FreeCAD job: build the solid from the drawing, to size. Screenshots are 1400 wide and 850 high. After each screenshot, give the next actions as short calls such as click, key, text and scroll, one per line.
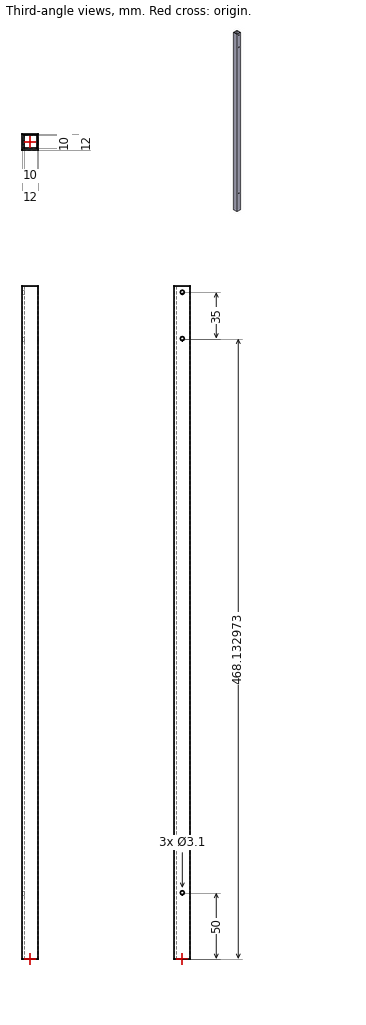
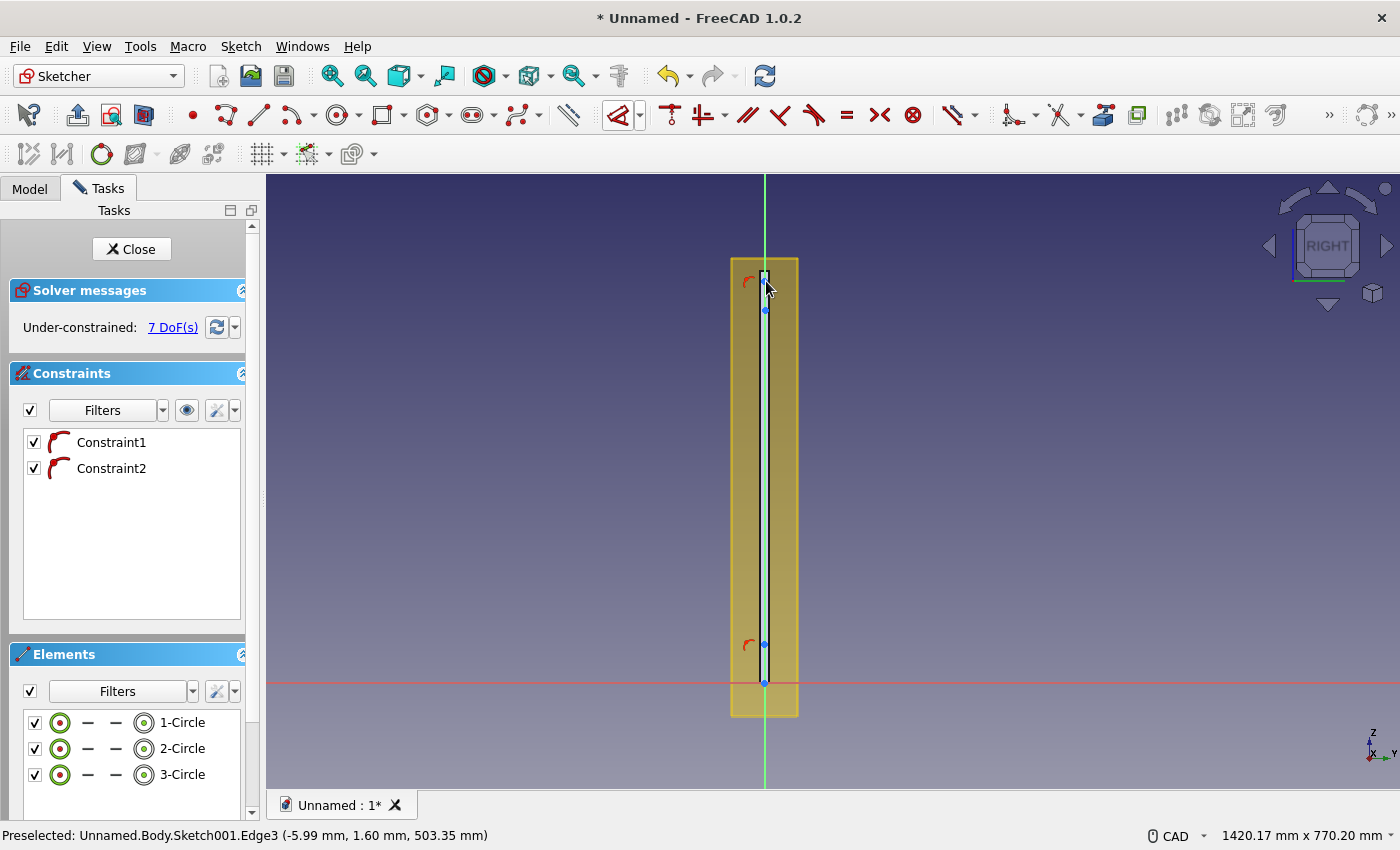
scroll(766, 643, up, 13)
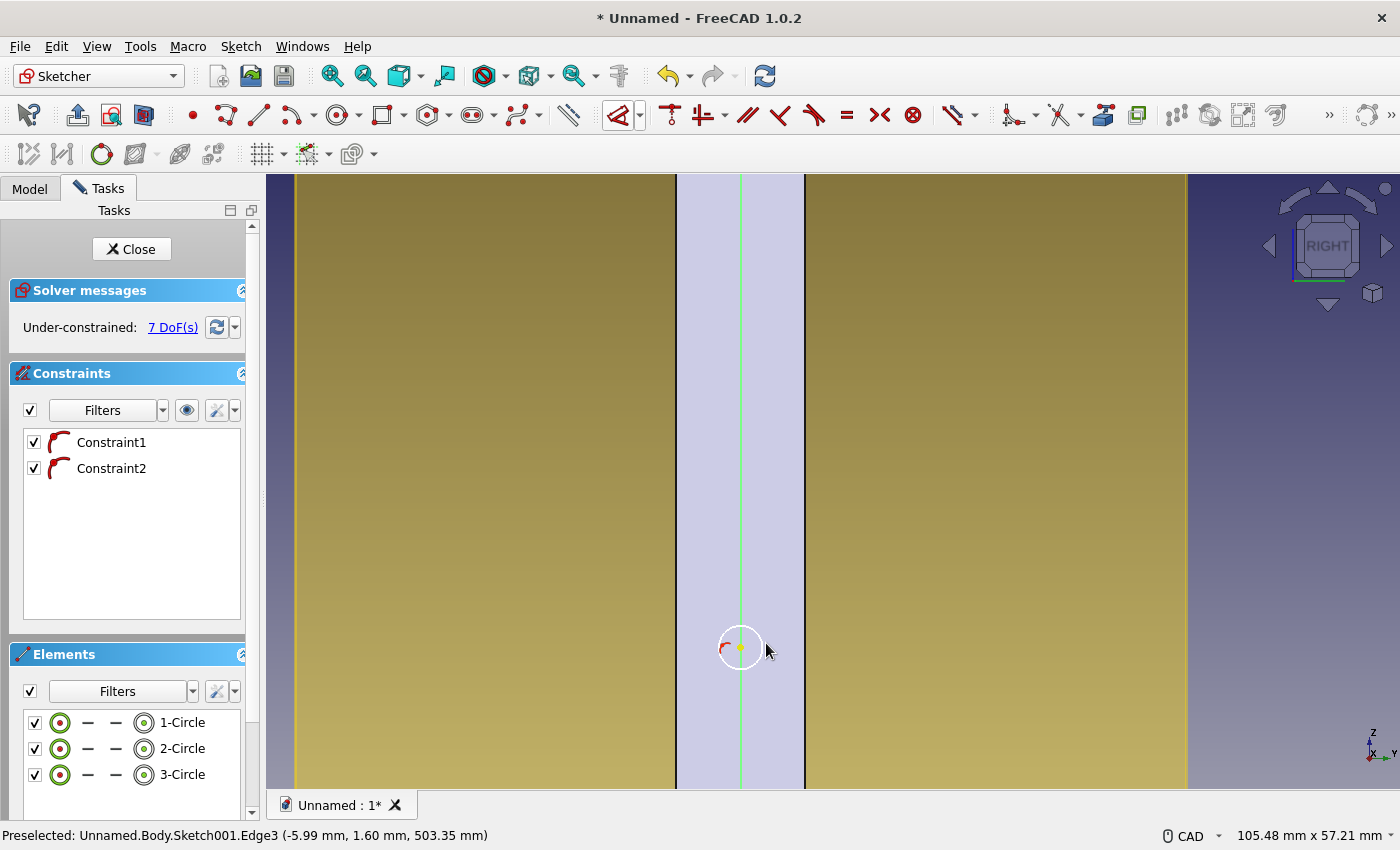
click(756, 632)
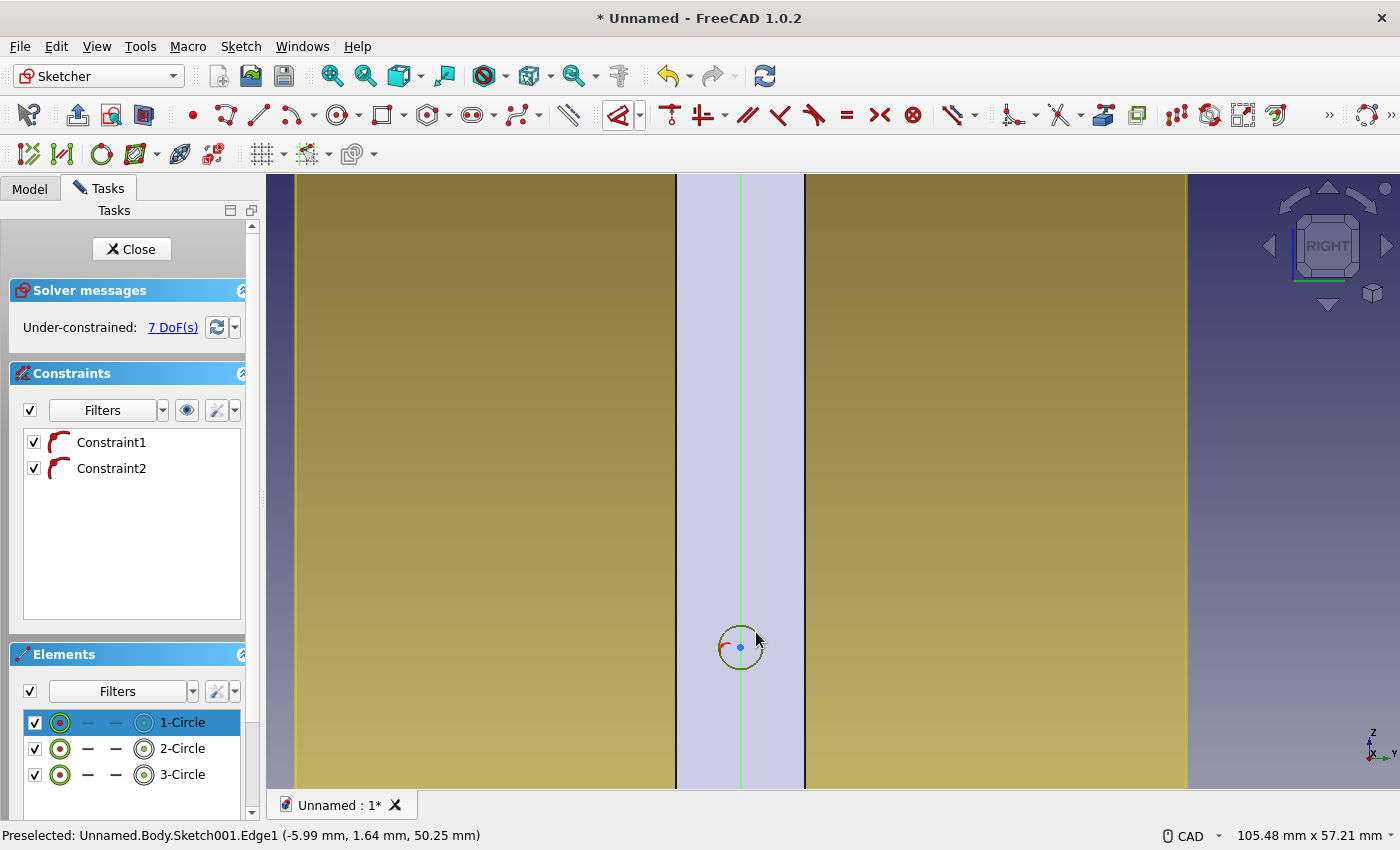
scroll(766, 644, down, 13)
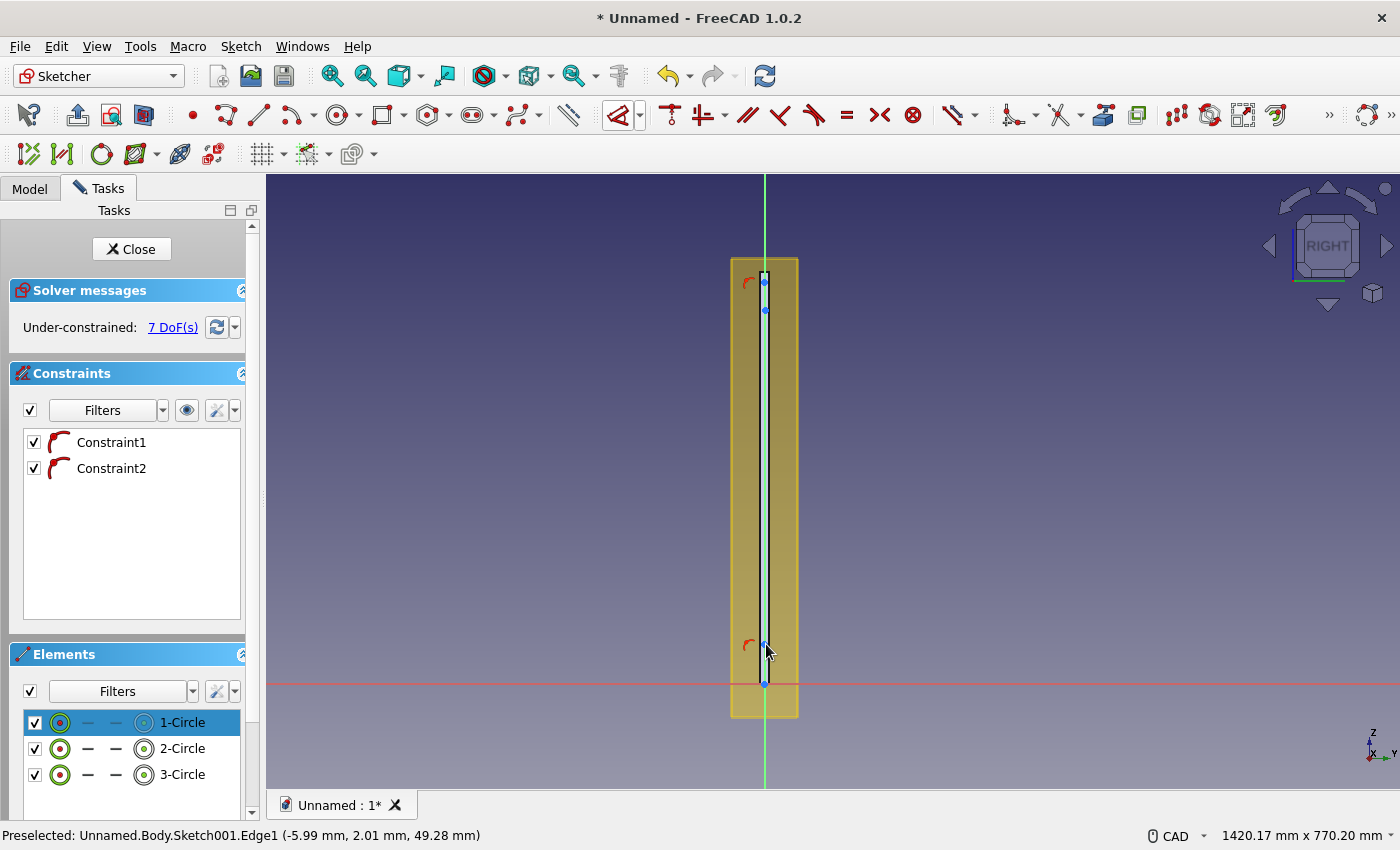
scroll(766, 310, up, 13)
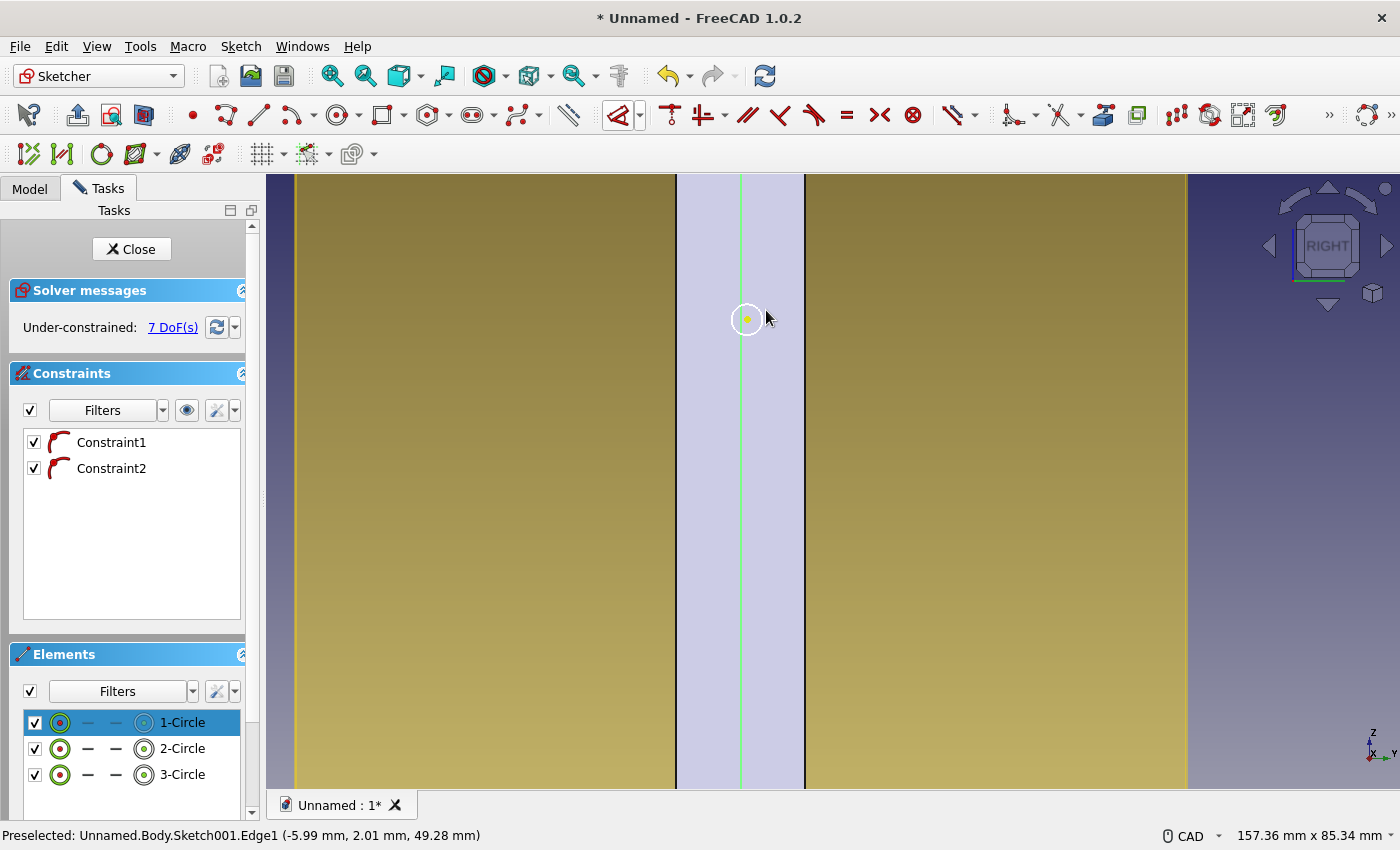
click(758, 309)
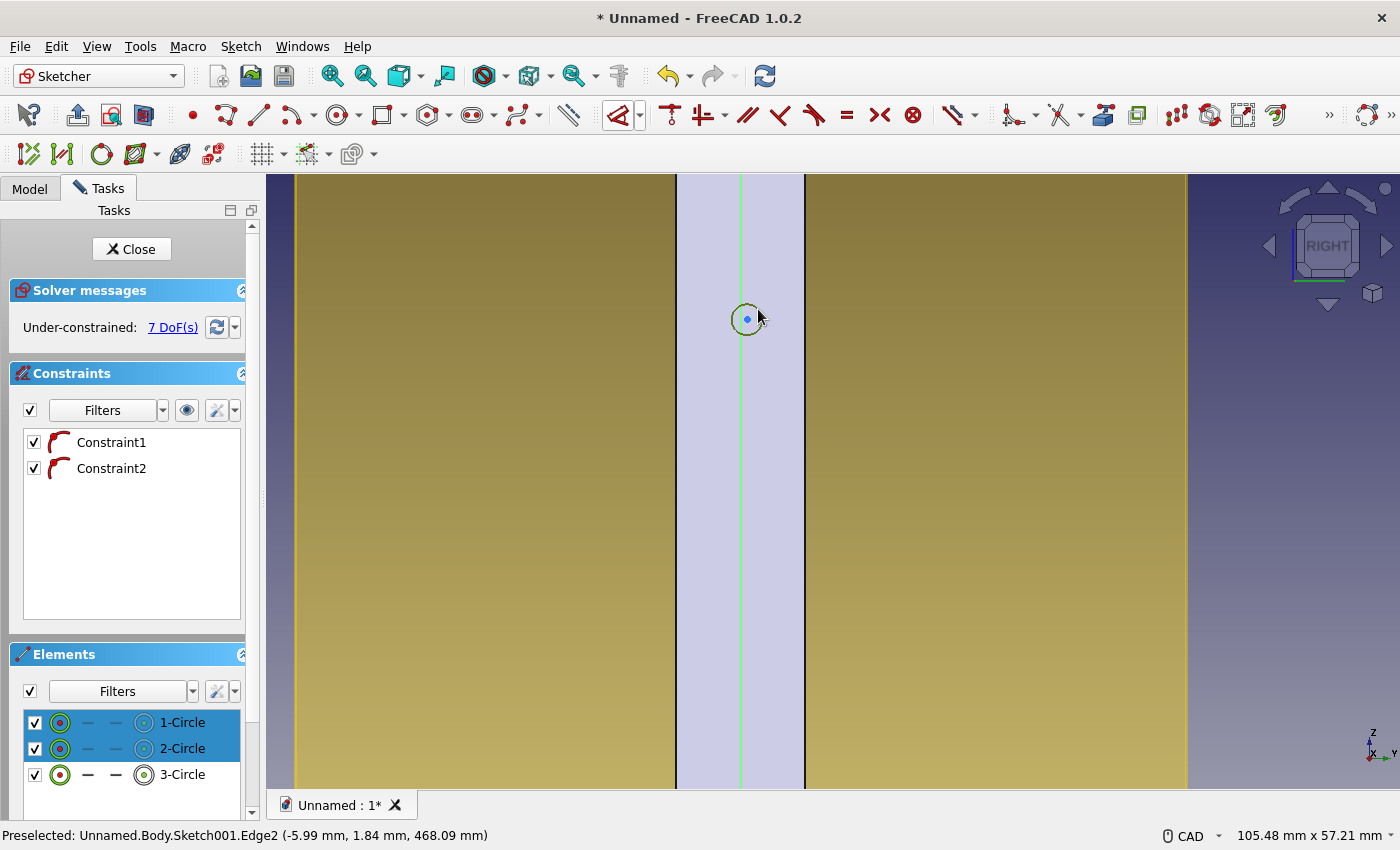
scroll(766, 309, down, 13)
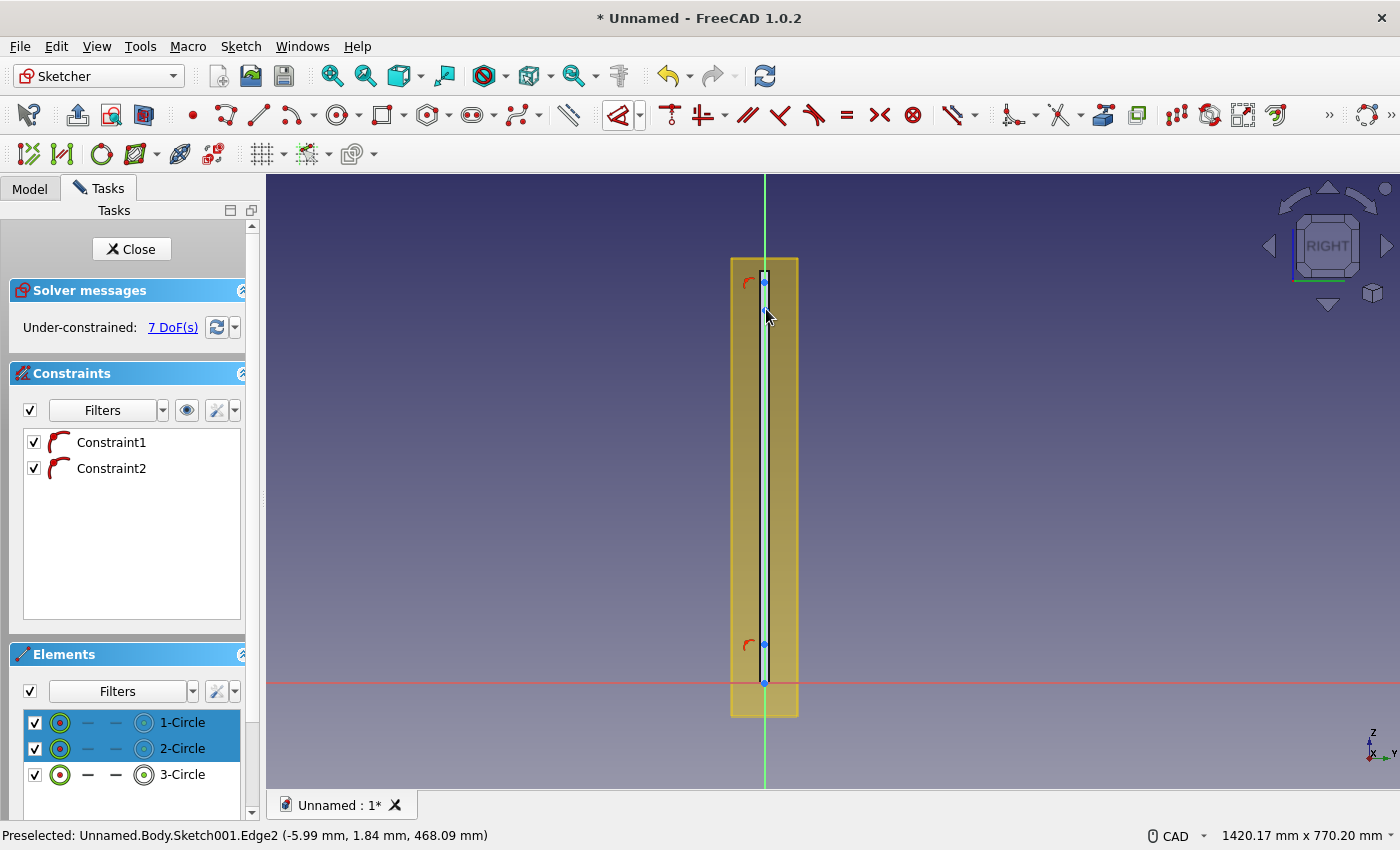
scroll(766, 281, up, 13)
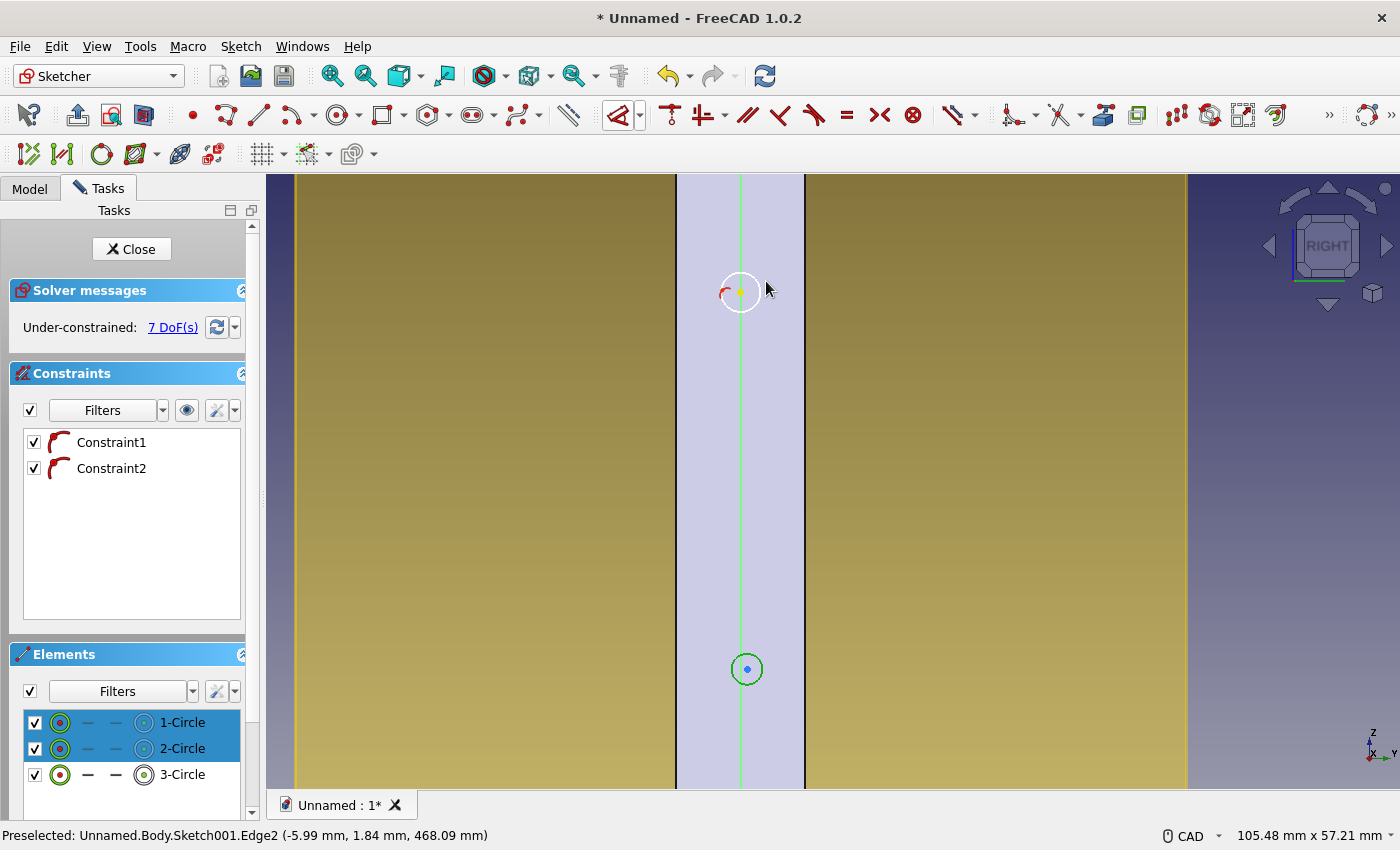
click(755, 278)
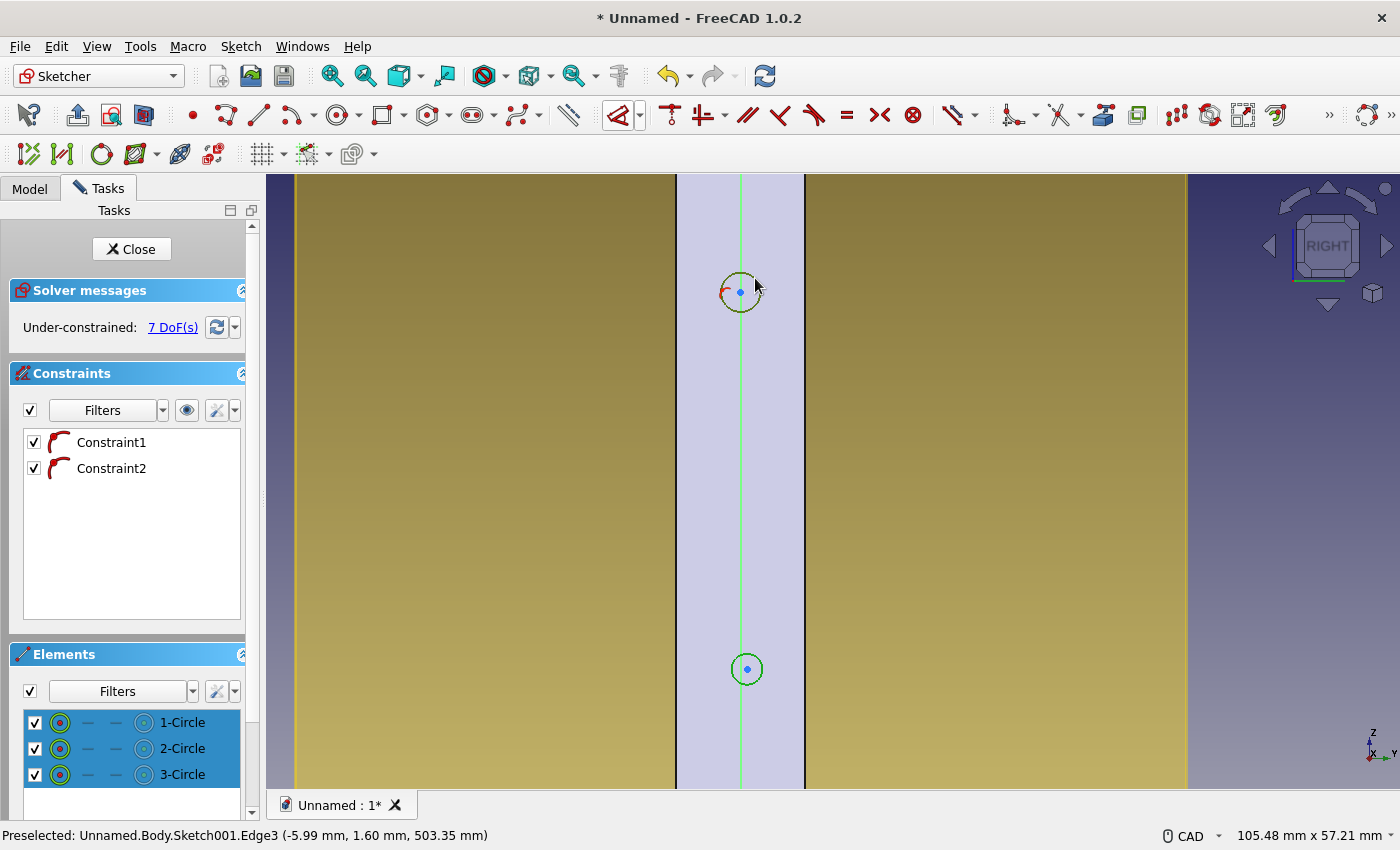
click(847, 116)